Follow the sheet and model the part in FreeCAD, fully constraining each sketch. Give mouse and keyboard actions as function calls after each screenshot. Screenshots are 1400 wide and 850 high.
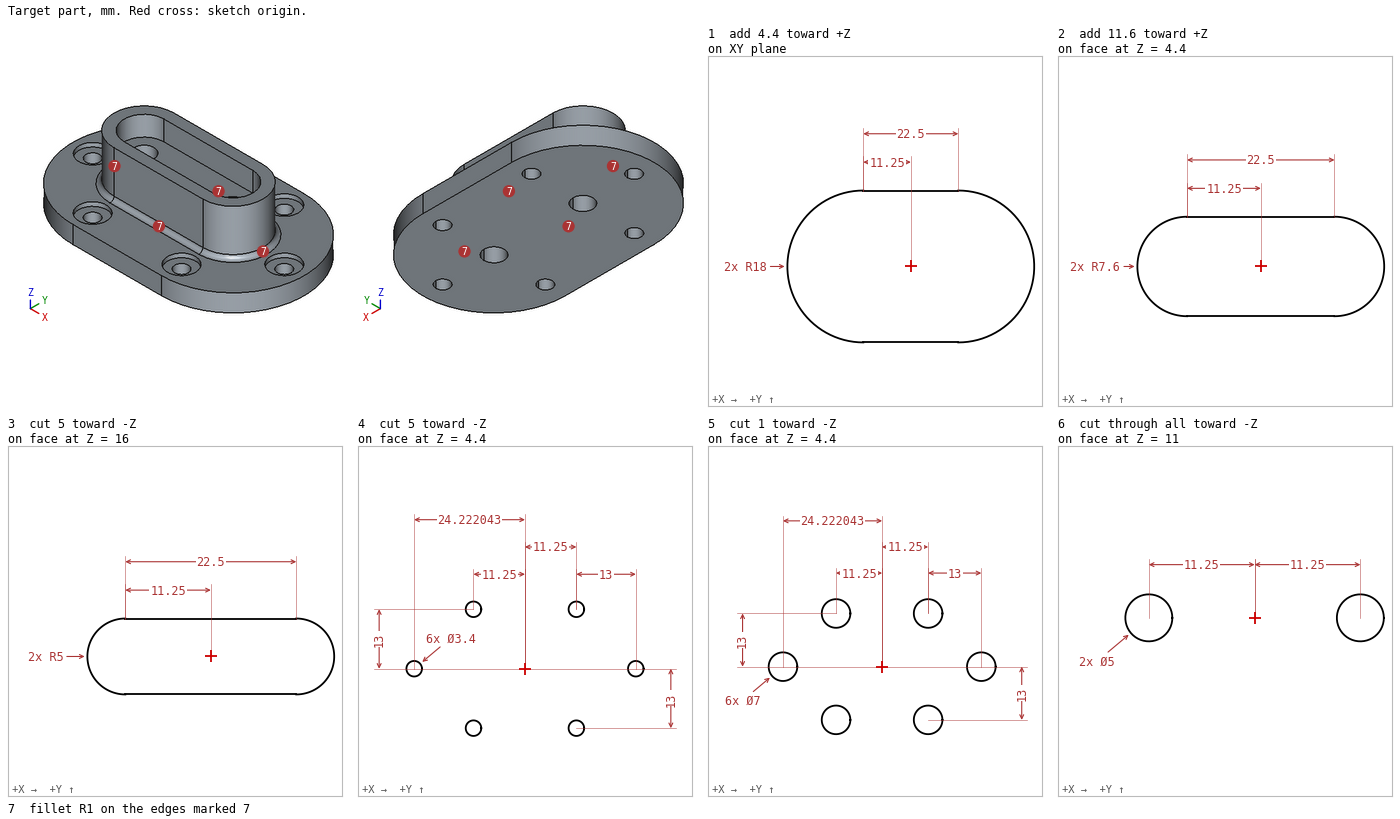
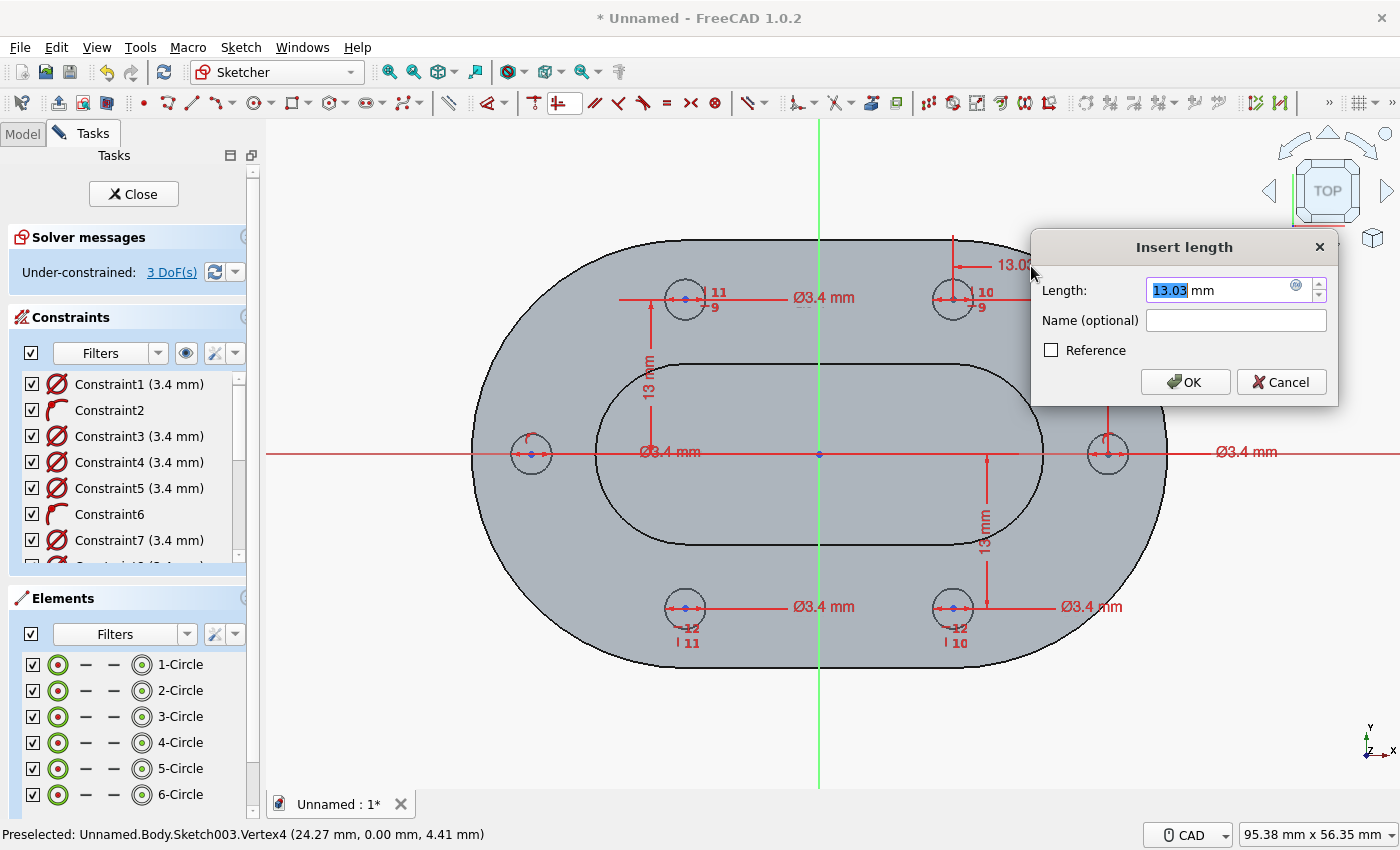
text(13)
key(Return)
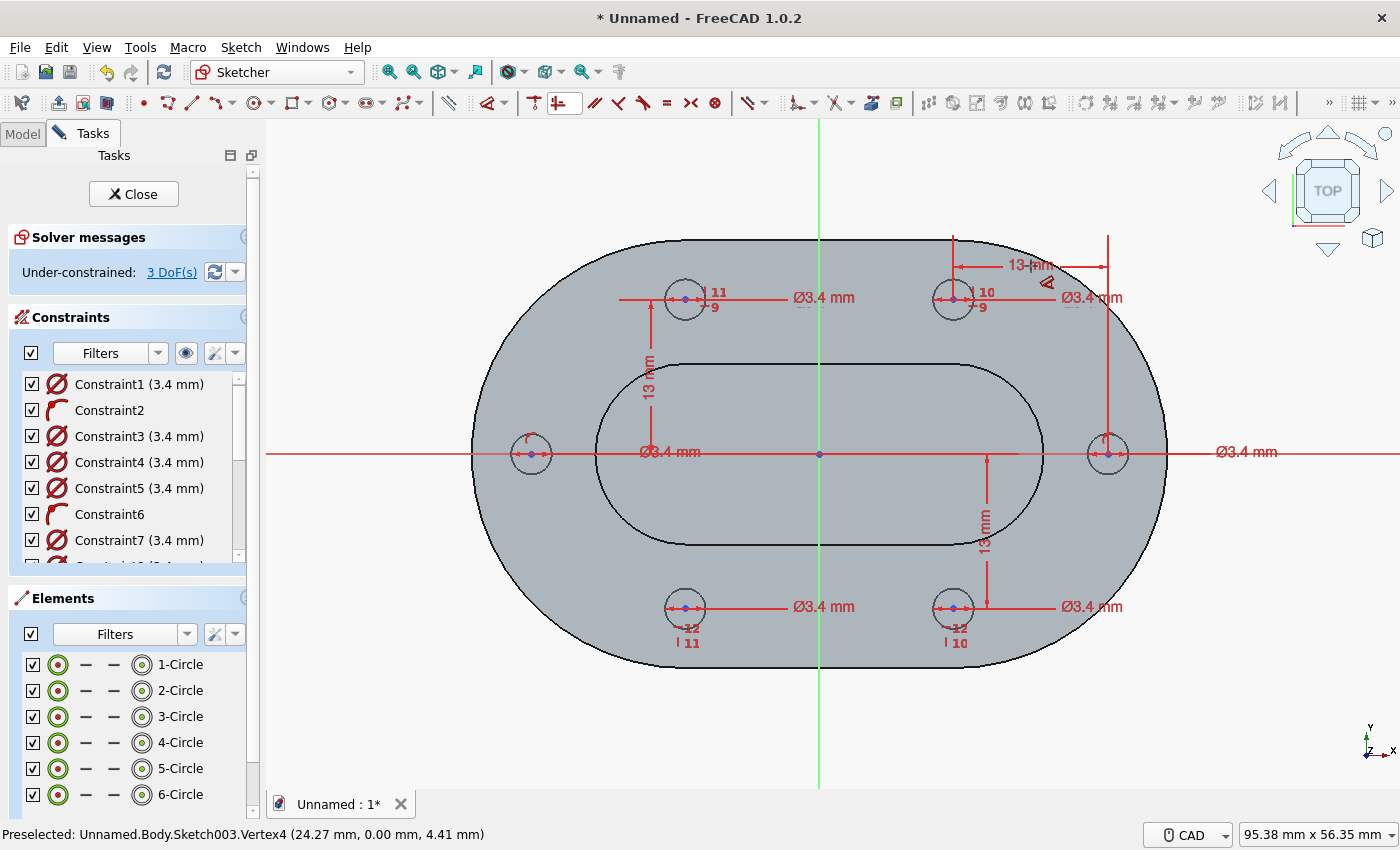
click(685, 300)
click(752, 266)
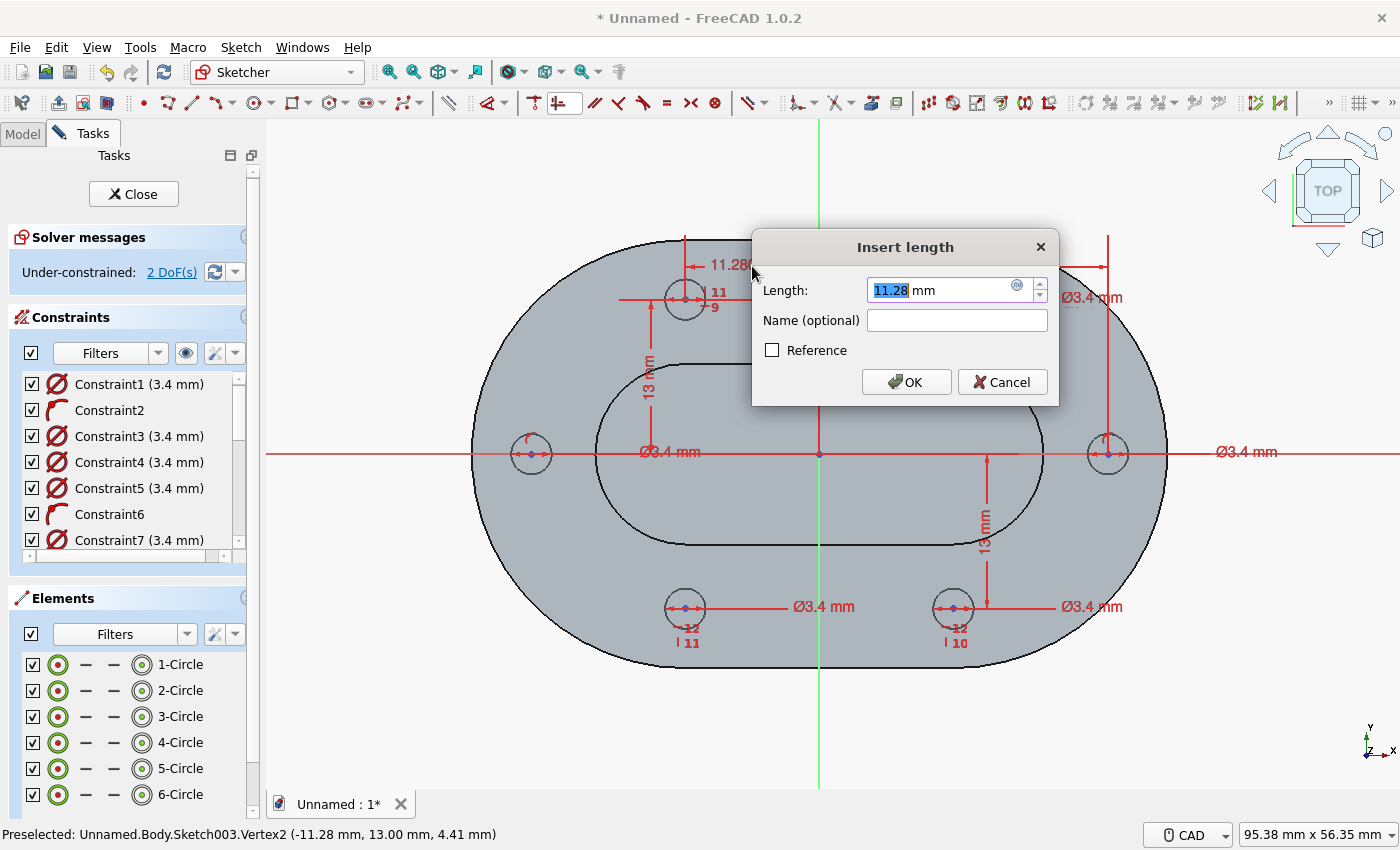
text(11.25)
key(Return)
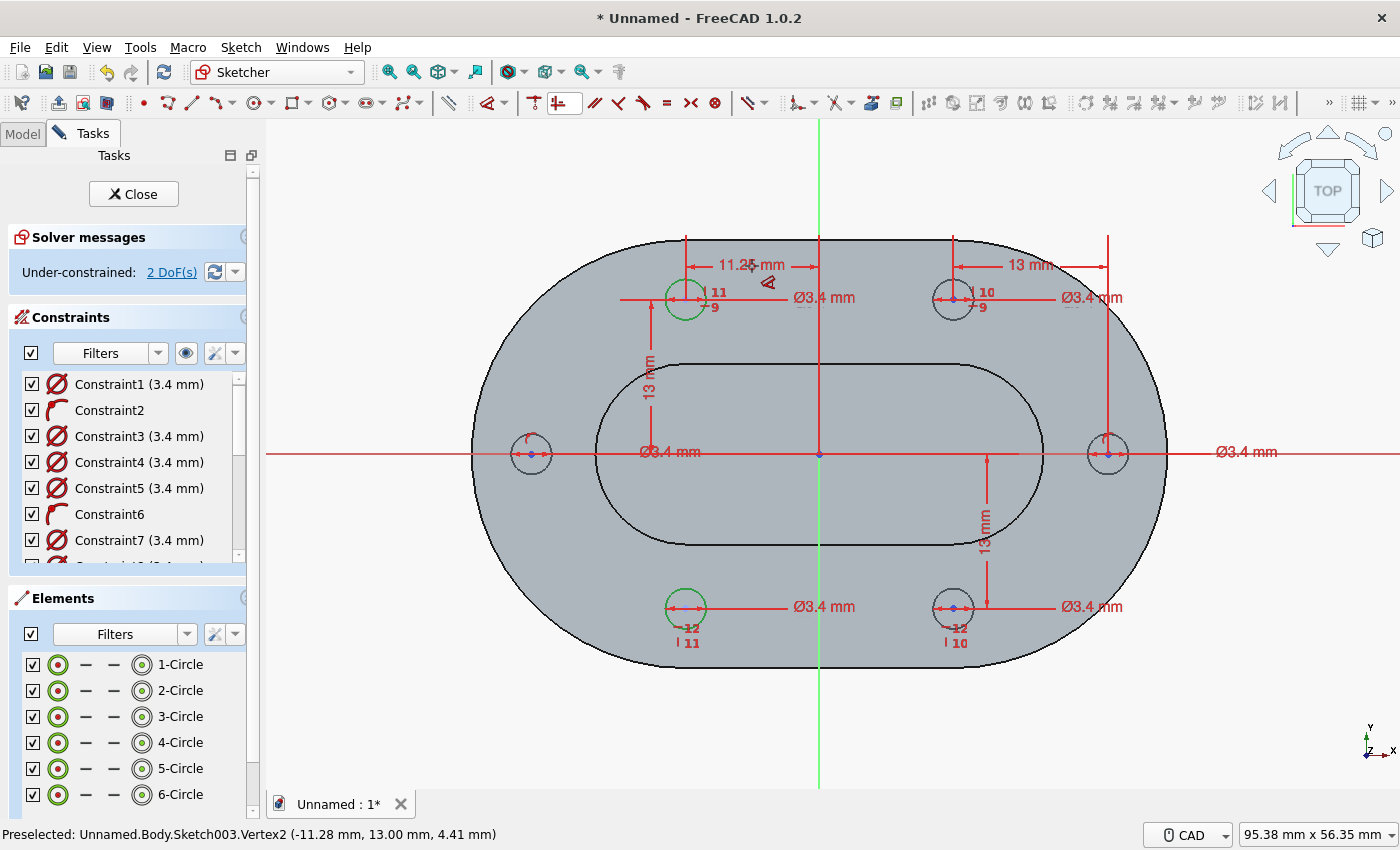
click(953, 300)
click(886, 266)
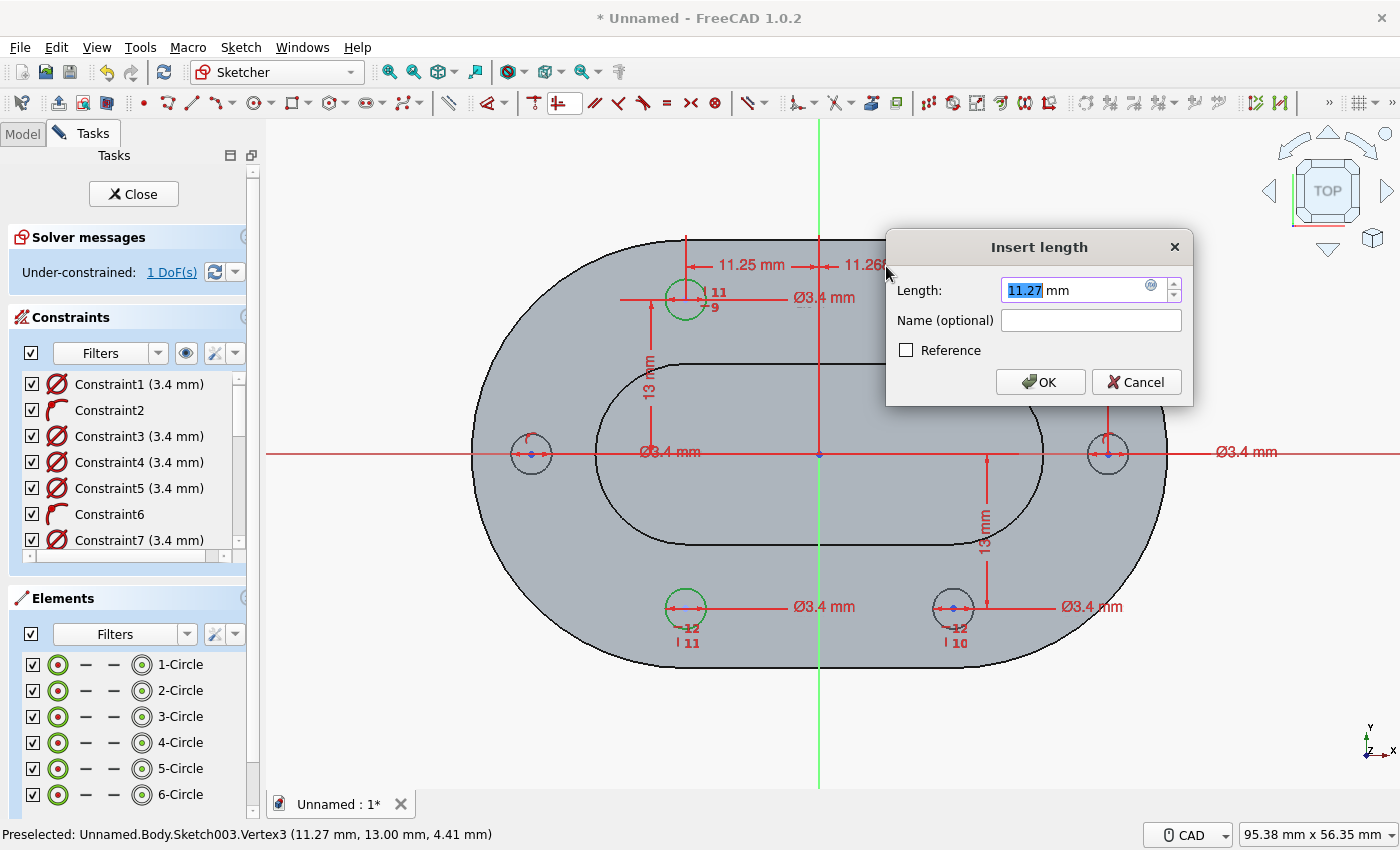
text(11.25)
key(Return)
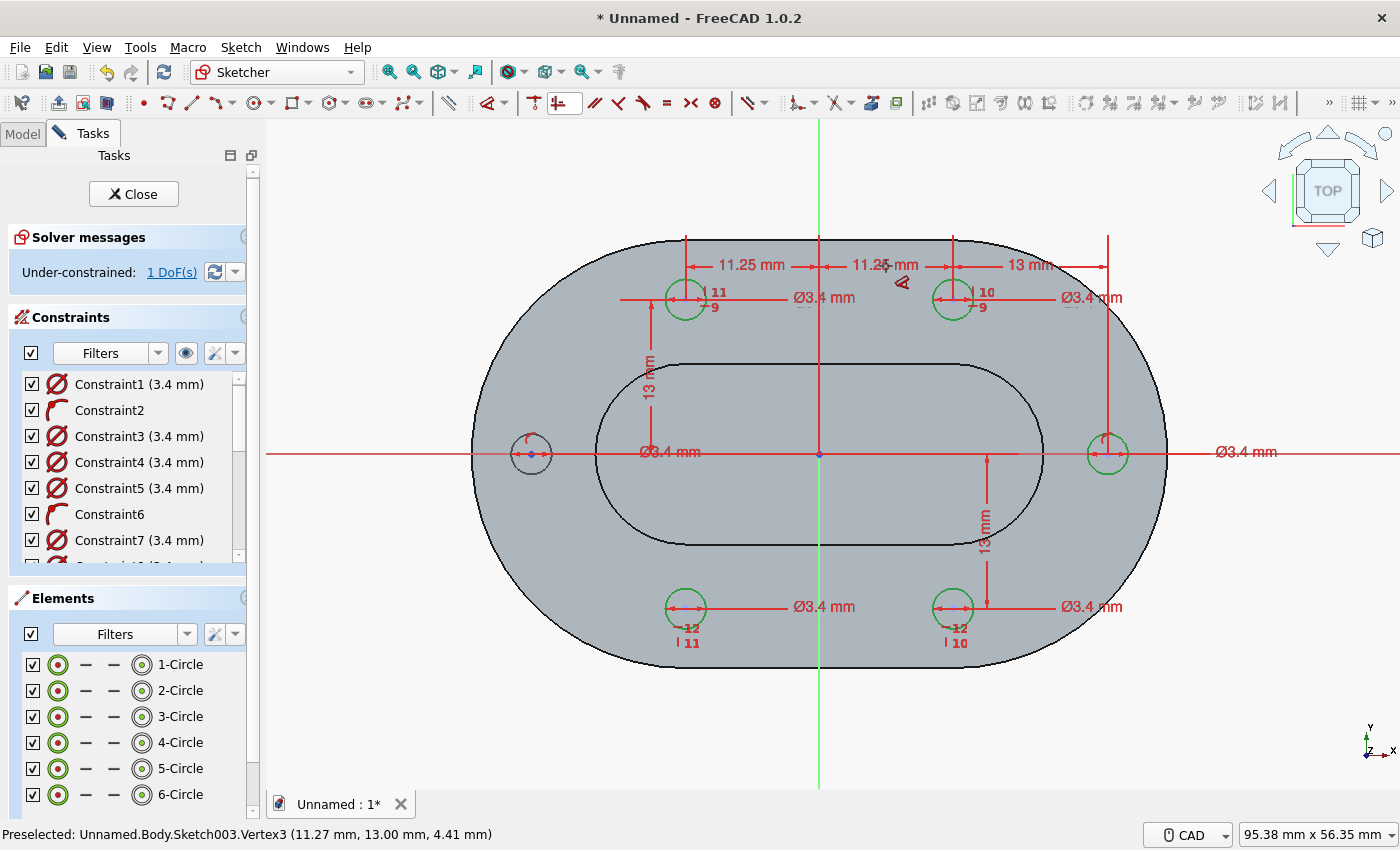
click(531, 454)
click(675, 488)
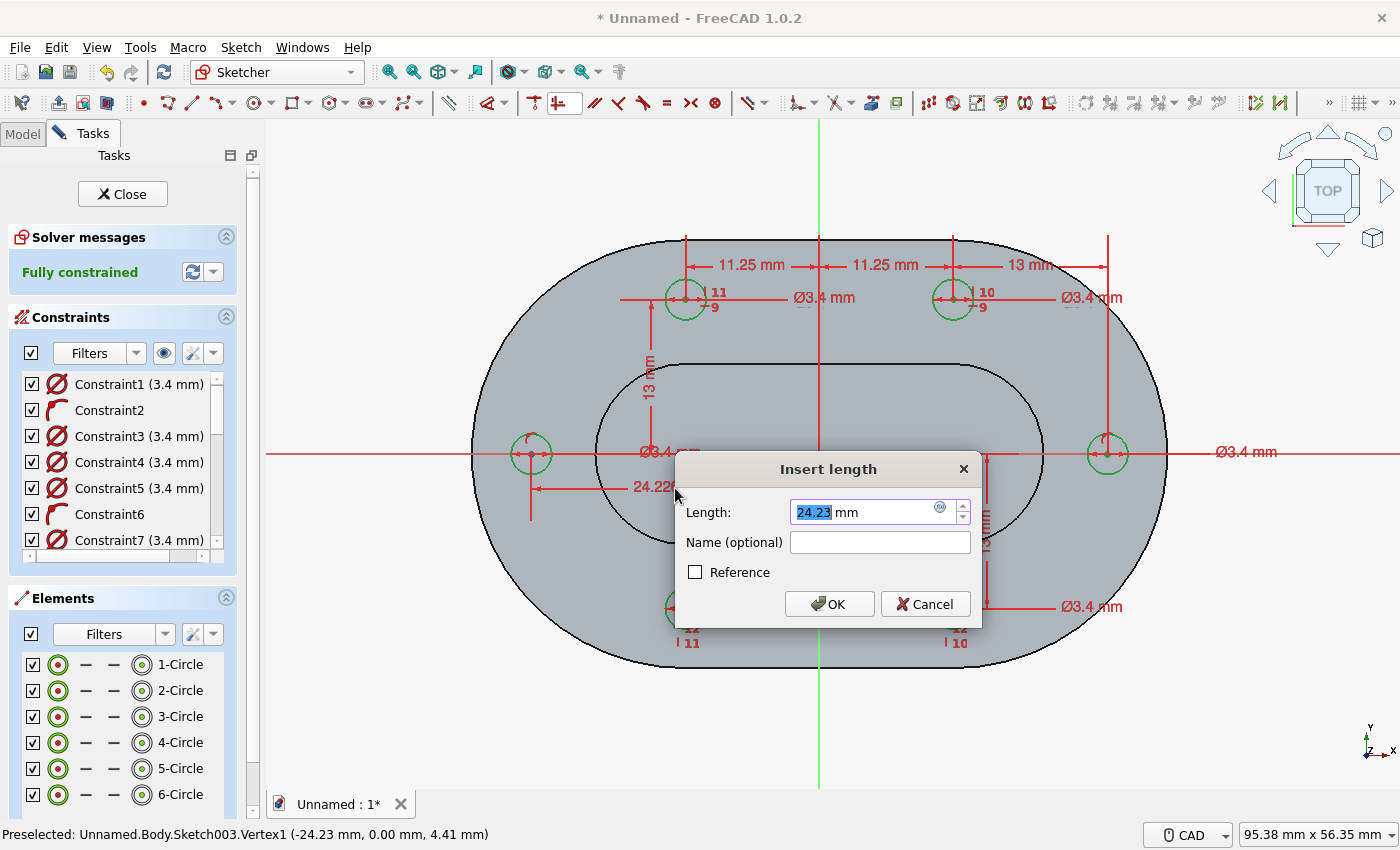
text(24.222043)
key(Return)
key(Escape)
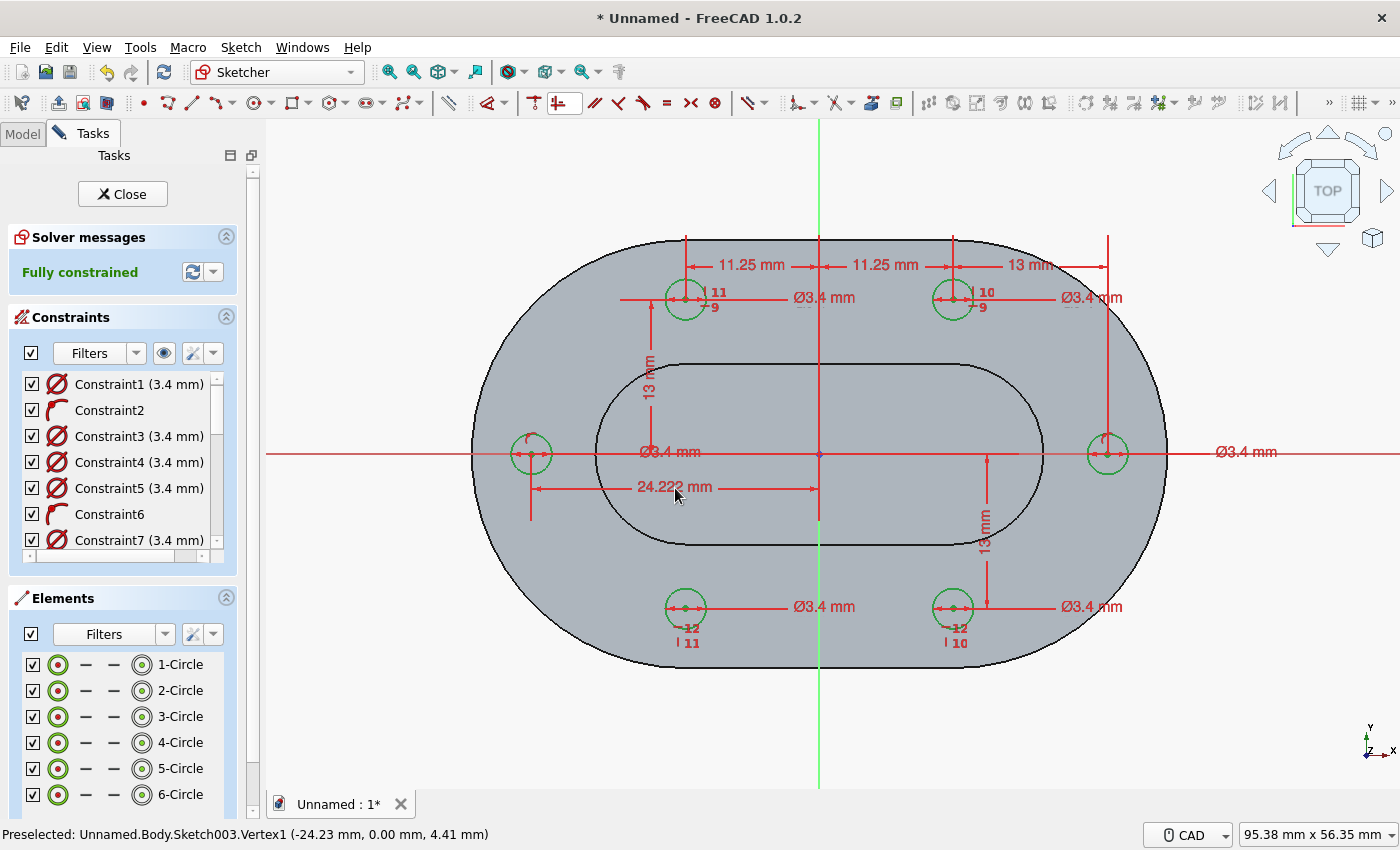
click(123, 194)